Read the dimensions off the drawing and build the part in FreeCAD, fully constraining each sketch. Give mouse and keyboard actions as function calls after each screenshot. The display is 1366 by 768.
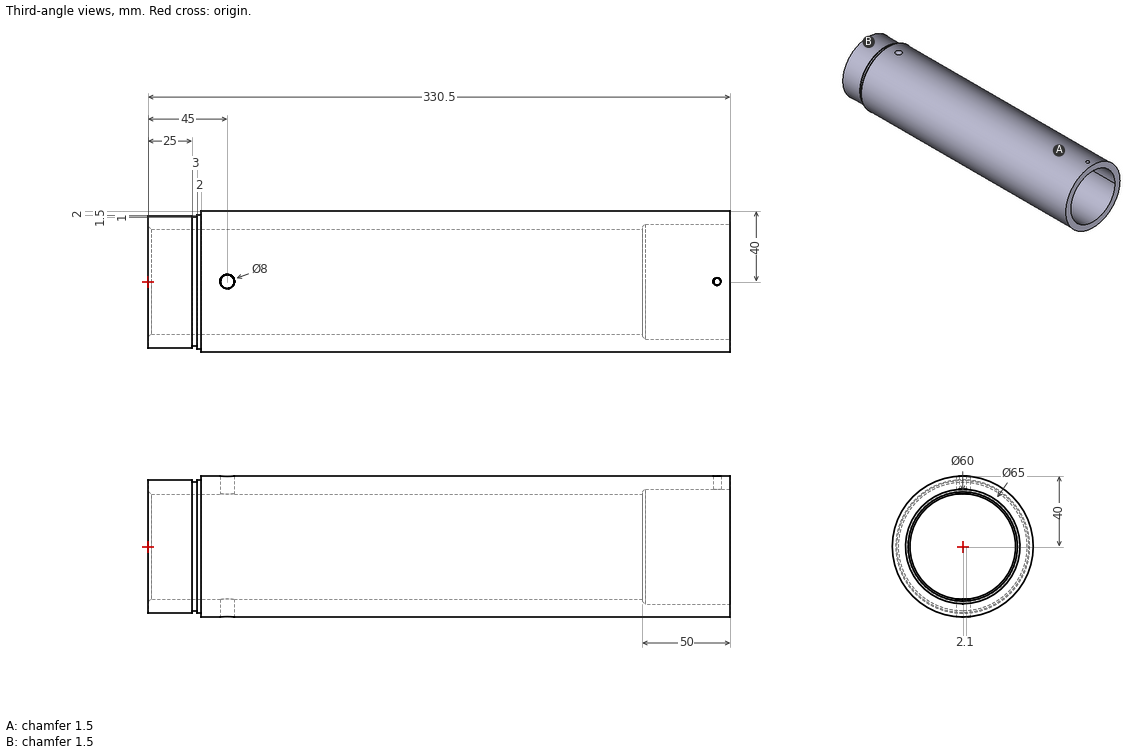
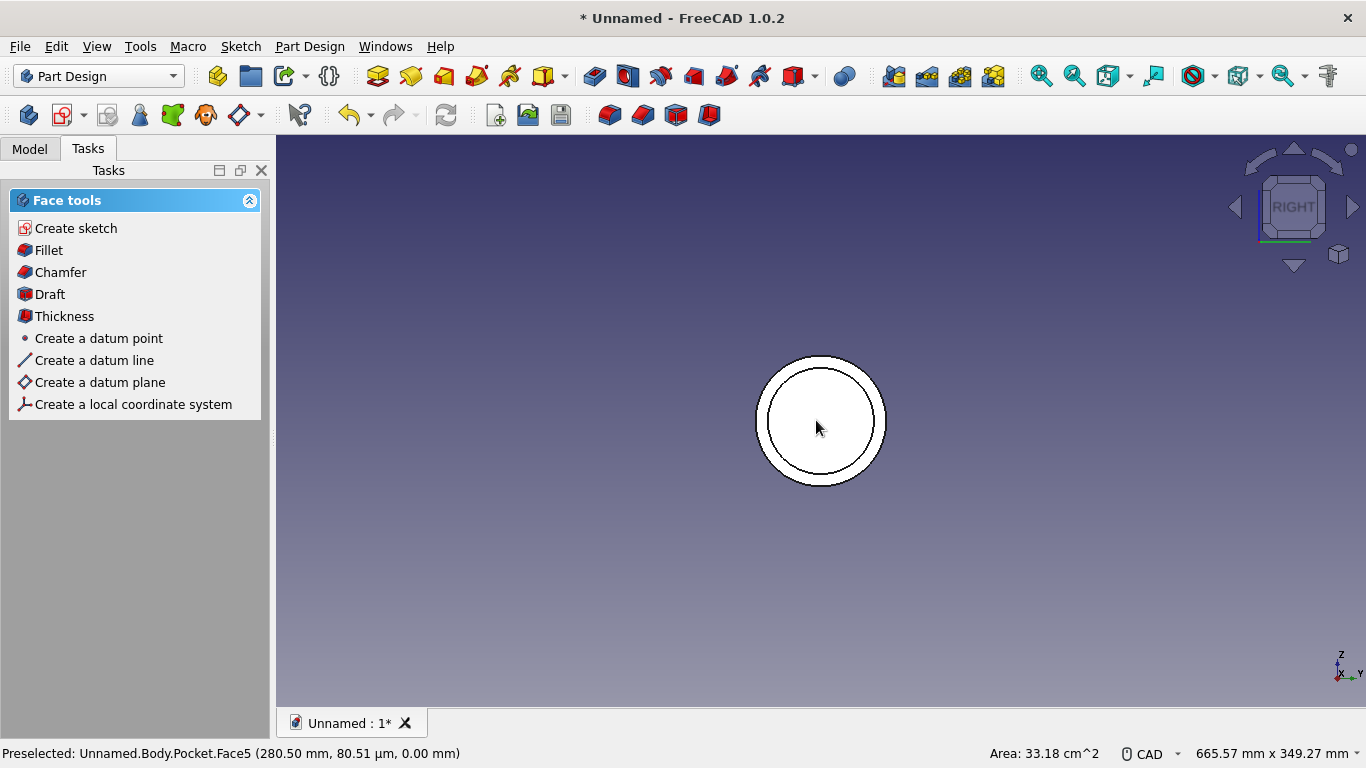
click(62, 116)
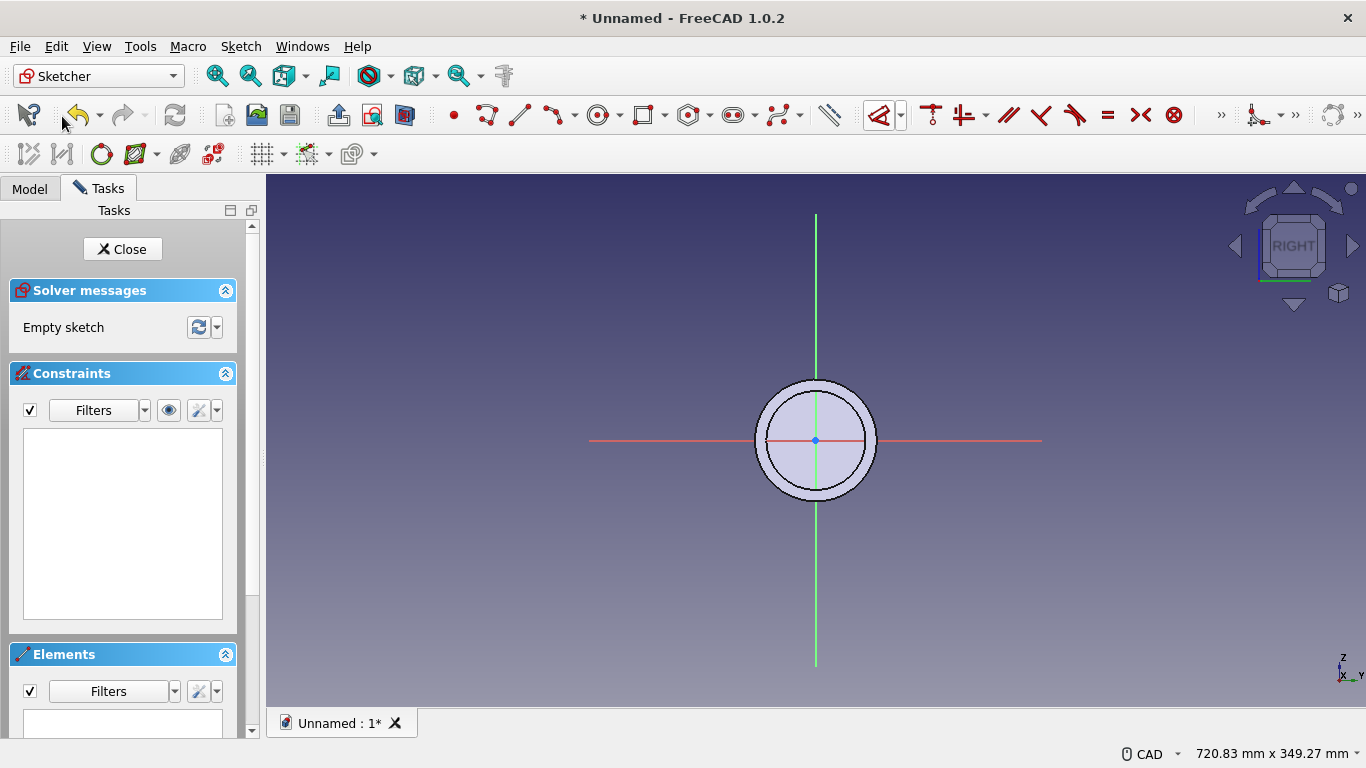
scroll(838, 440, up, 7)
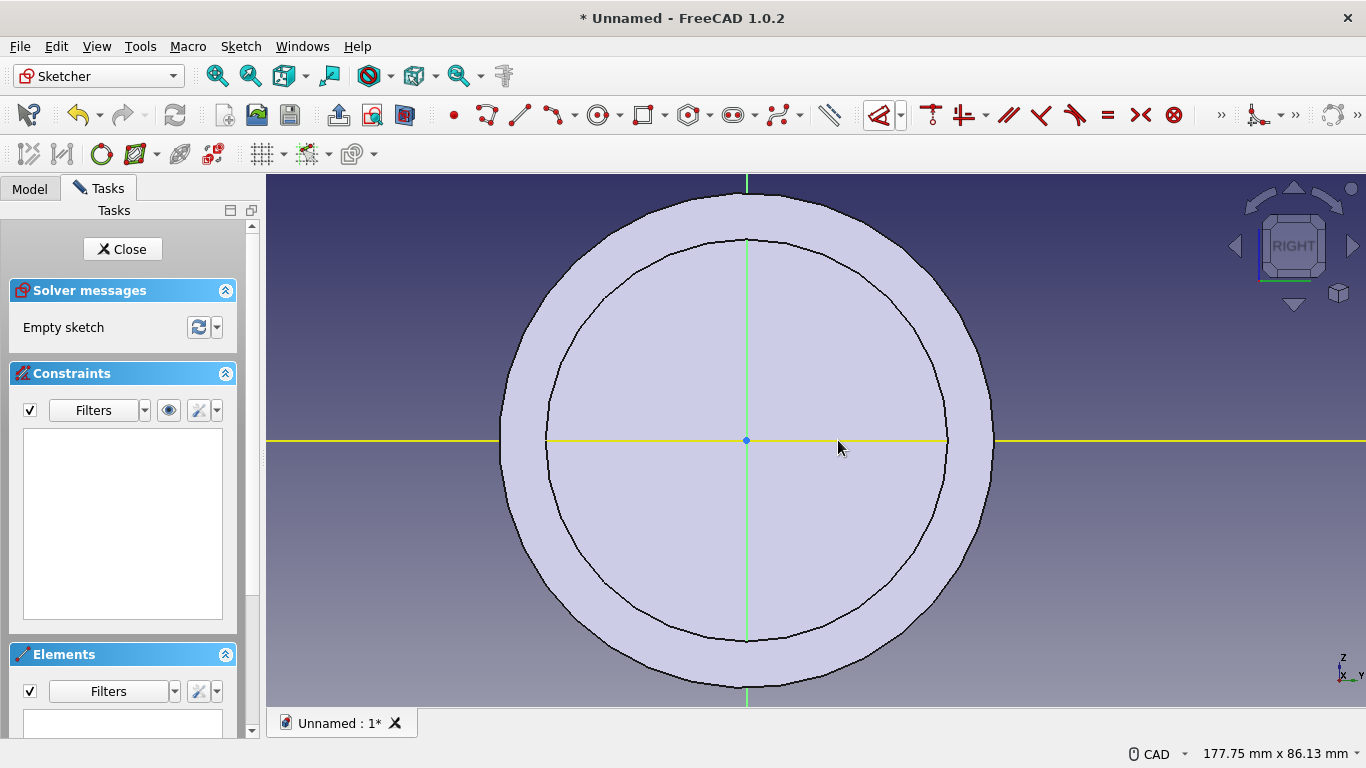
click(598, 116)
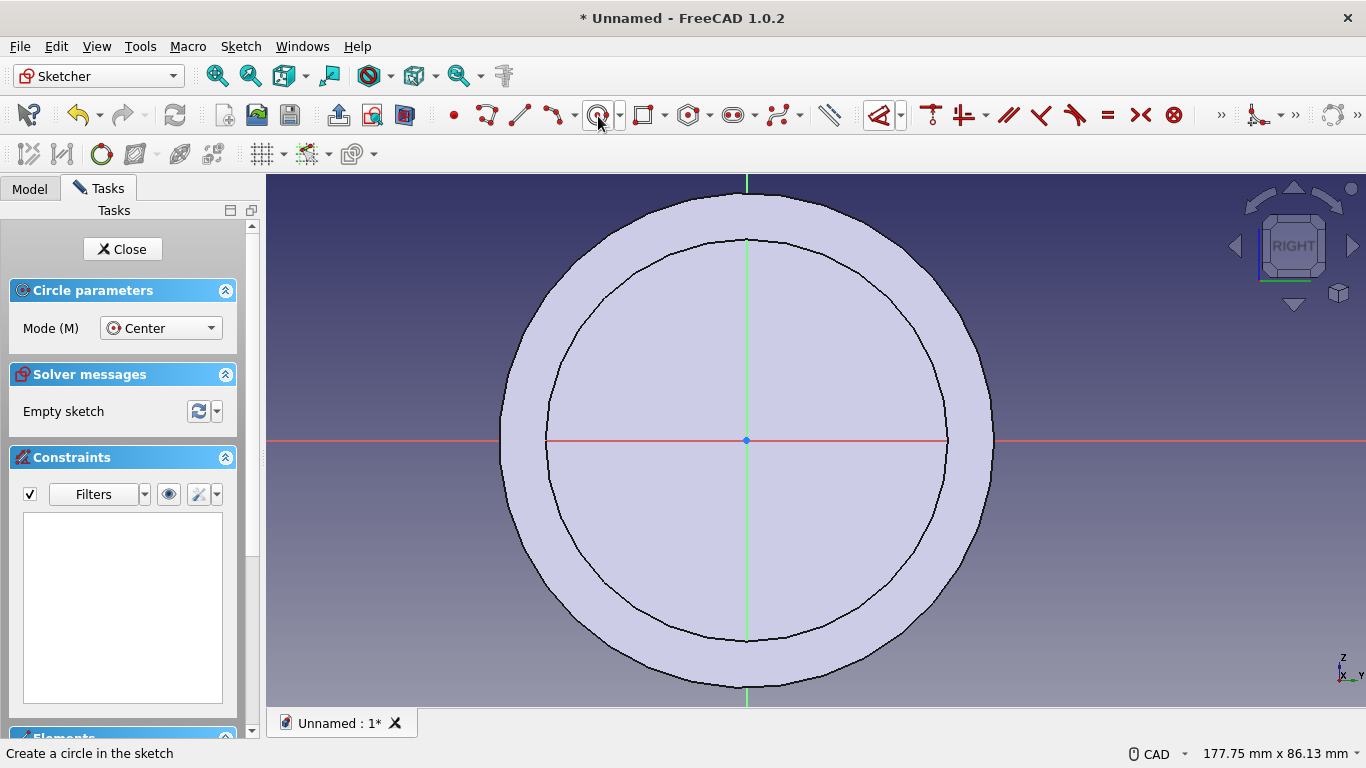
click(747, 440)
move(878, 309)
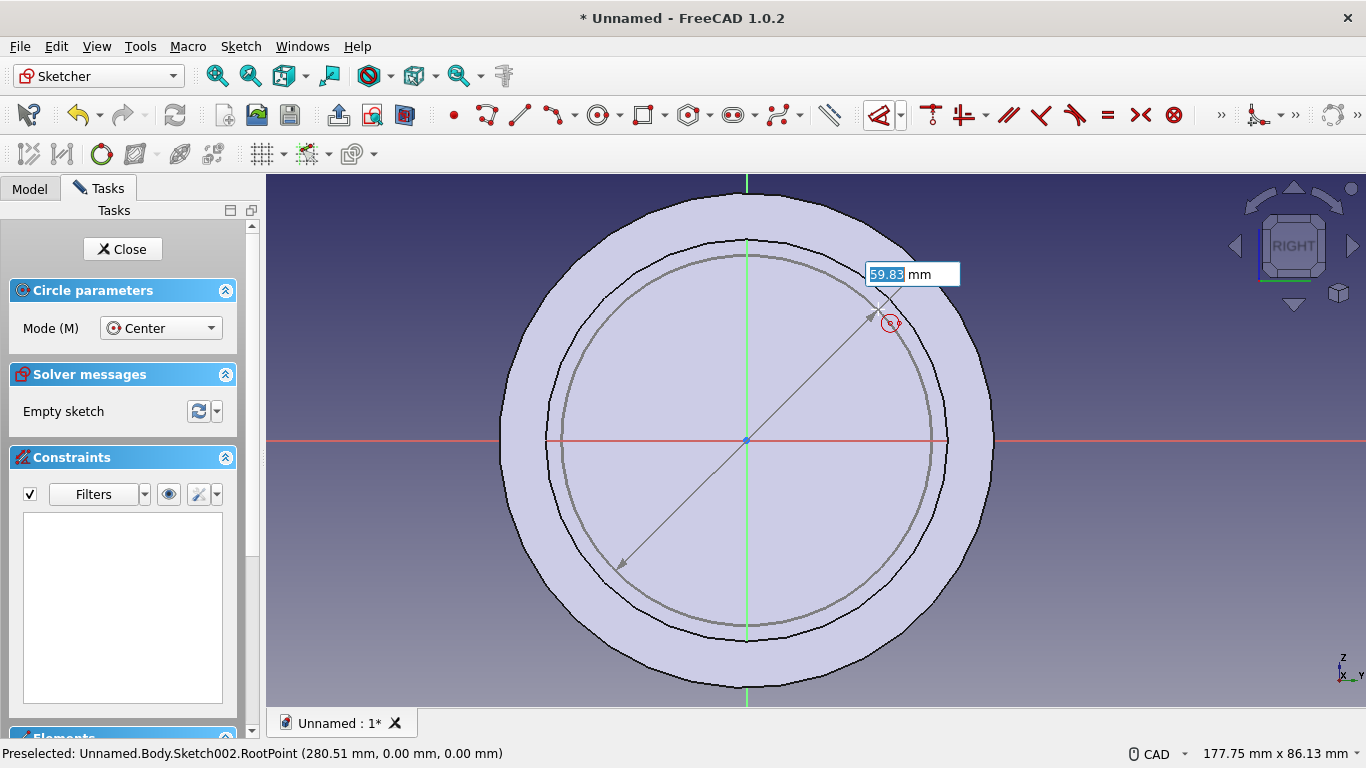
text(60)
key(Return)
key(Escape)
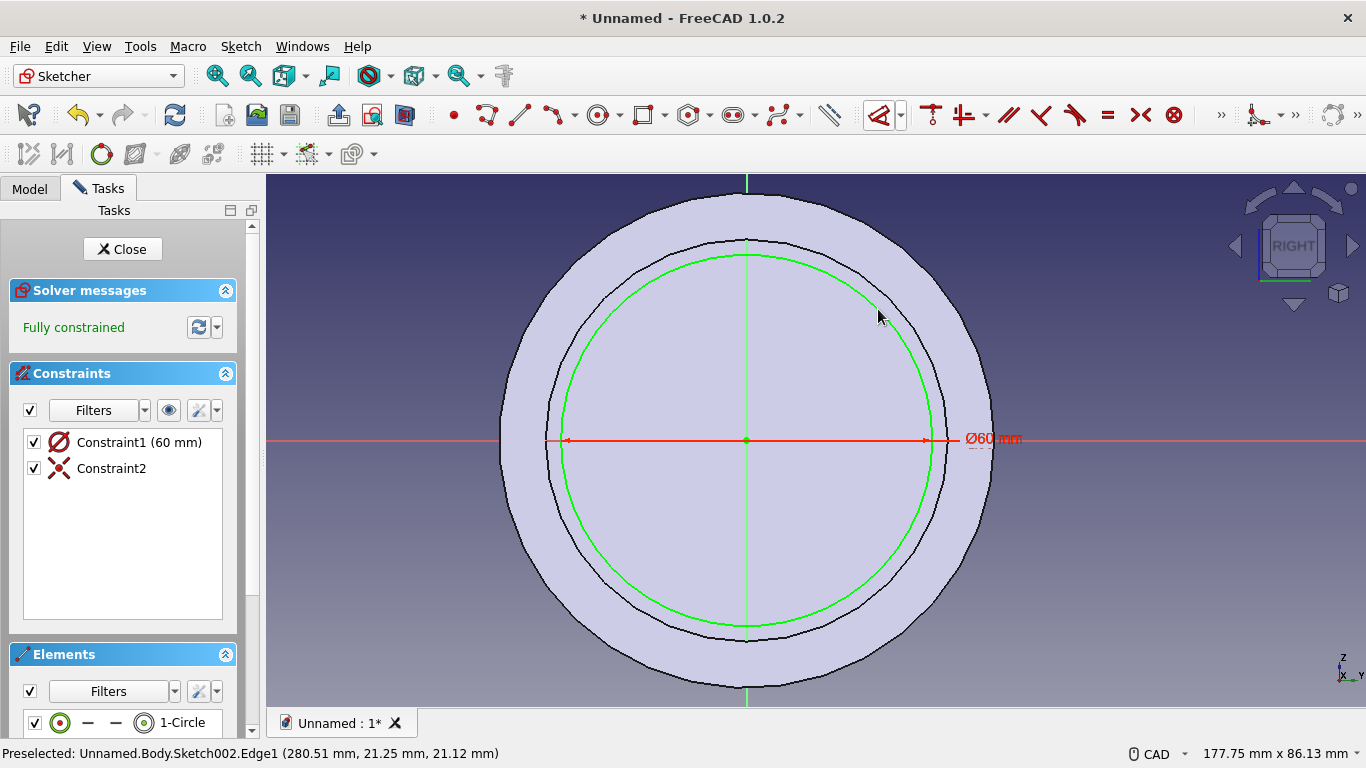
click(123, 249)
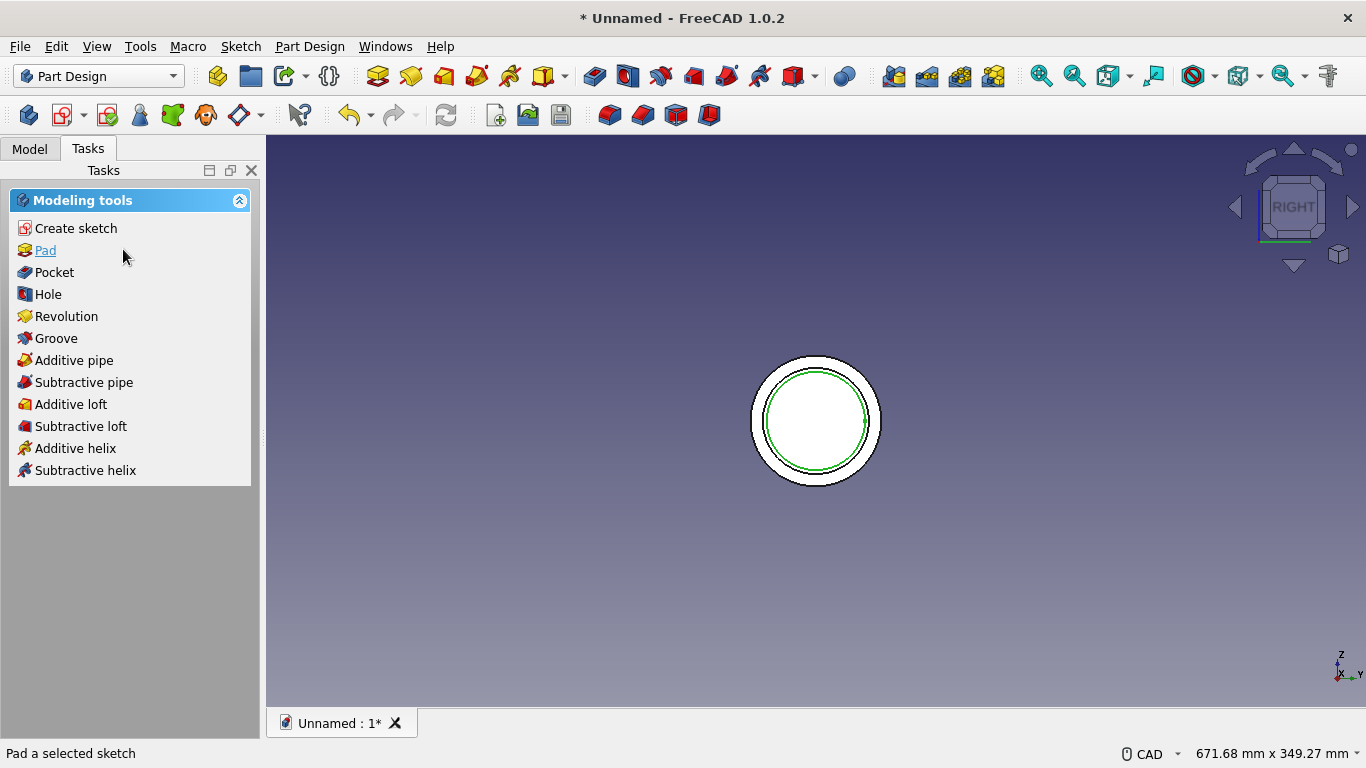
click(595, 76)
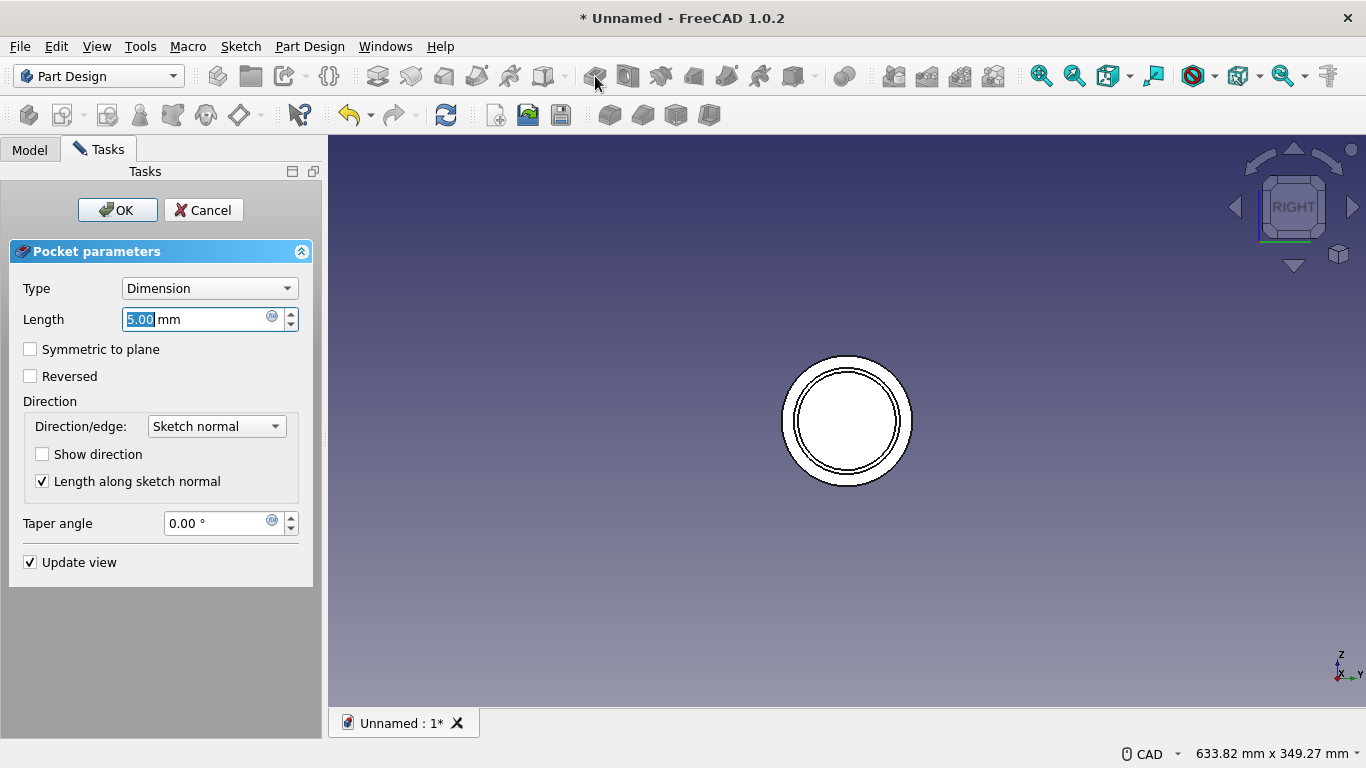
click(210, 288)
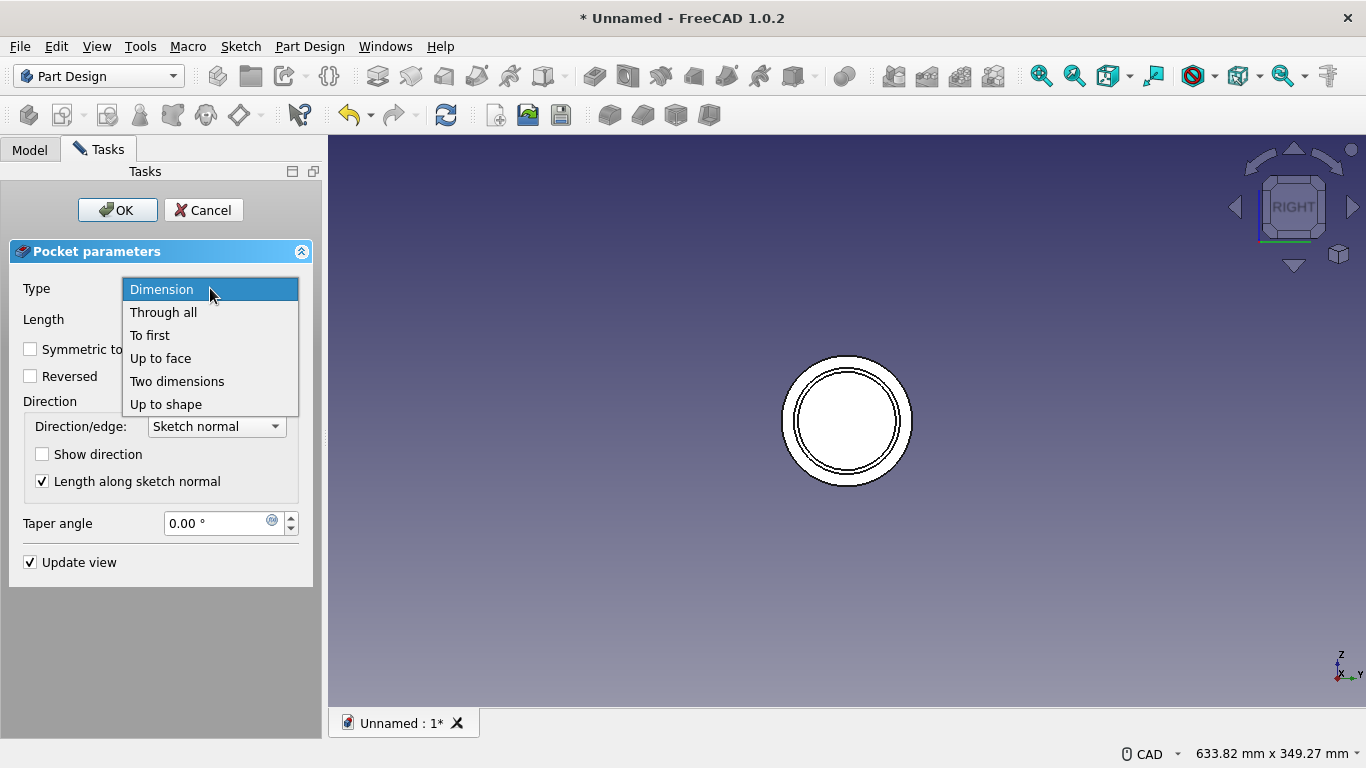
click(208, 312)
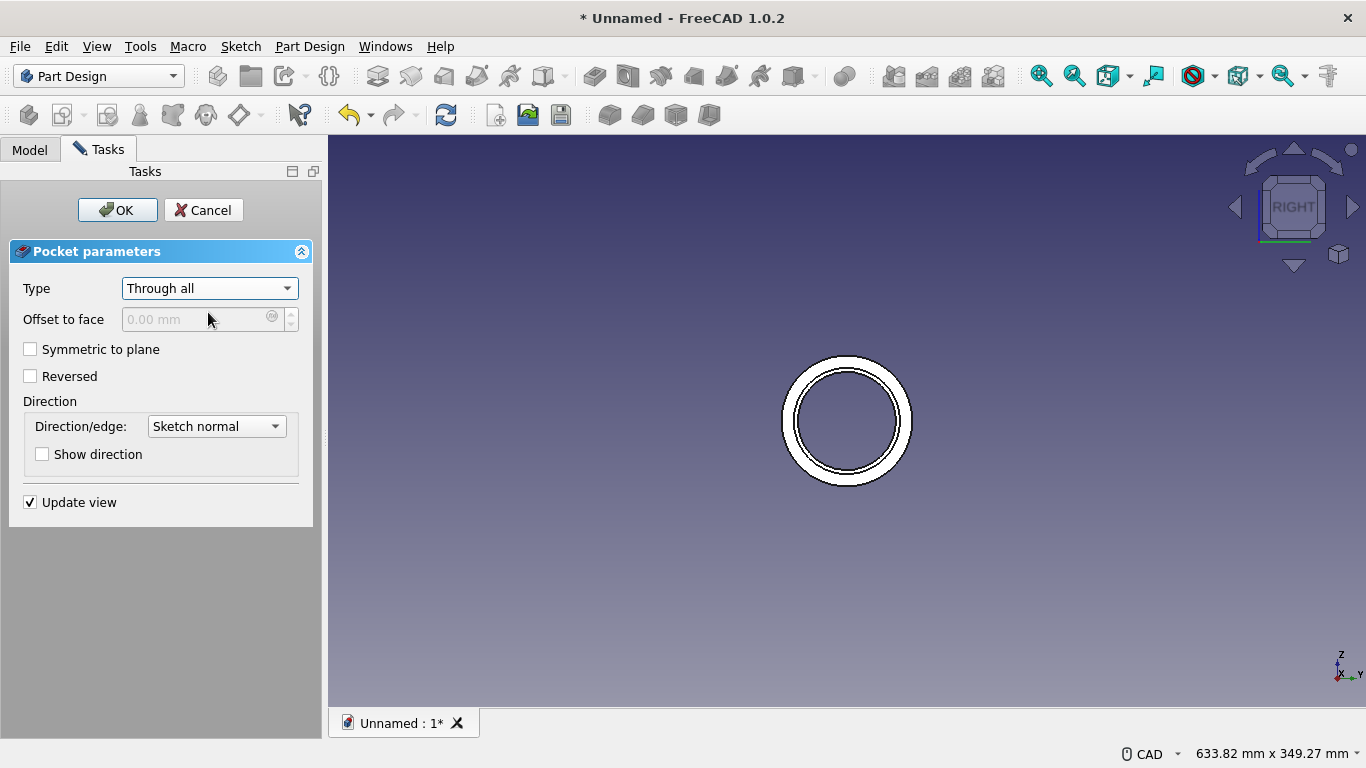
click(118, 210)